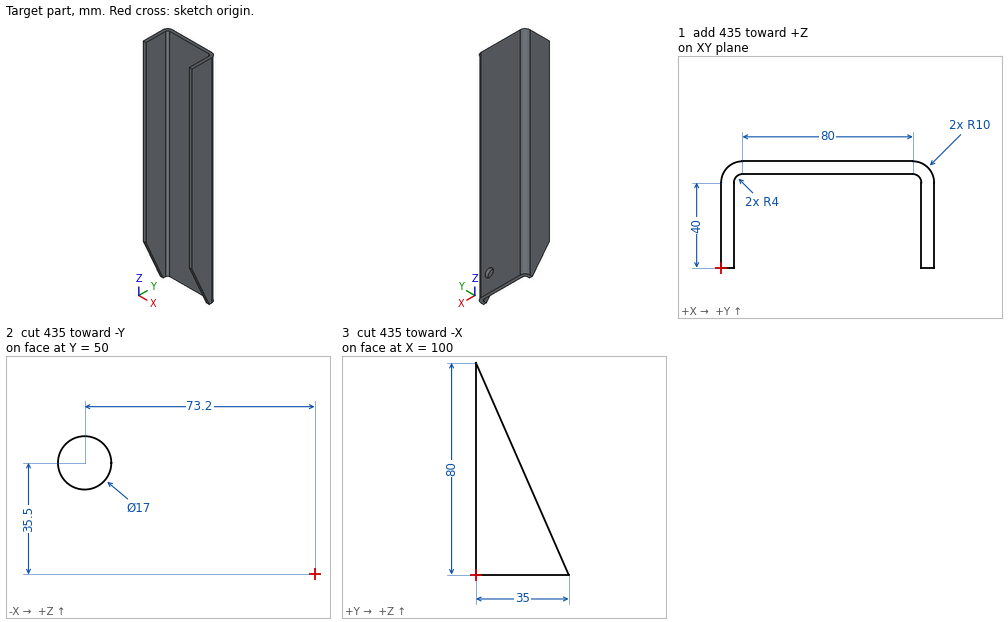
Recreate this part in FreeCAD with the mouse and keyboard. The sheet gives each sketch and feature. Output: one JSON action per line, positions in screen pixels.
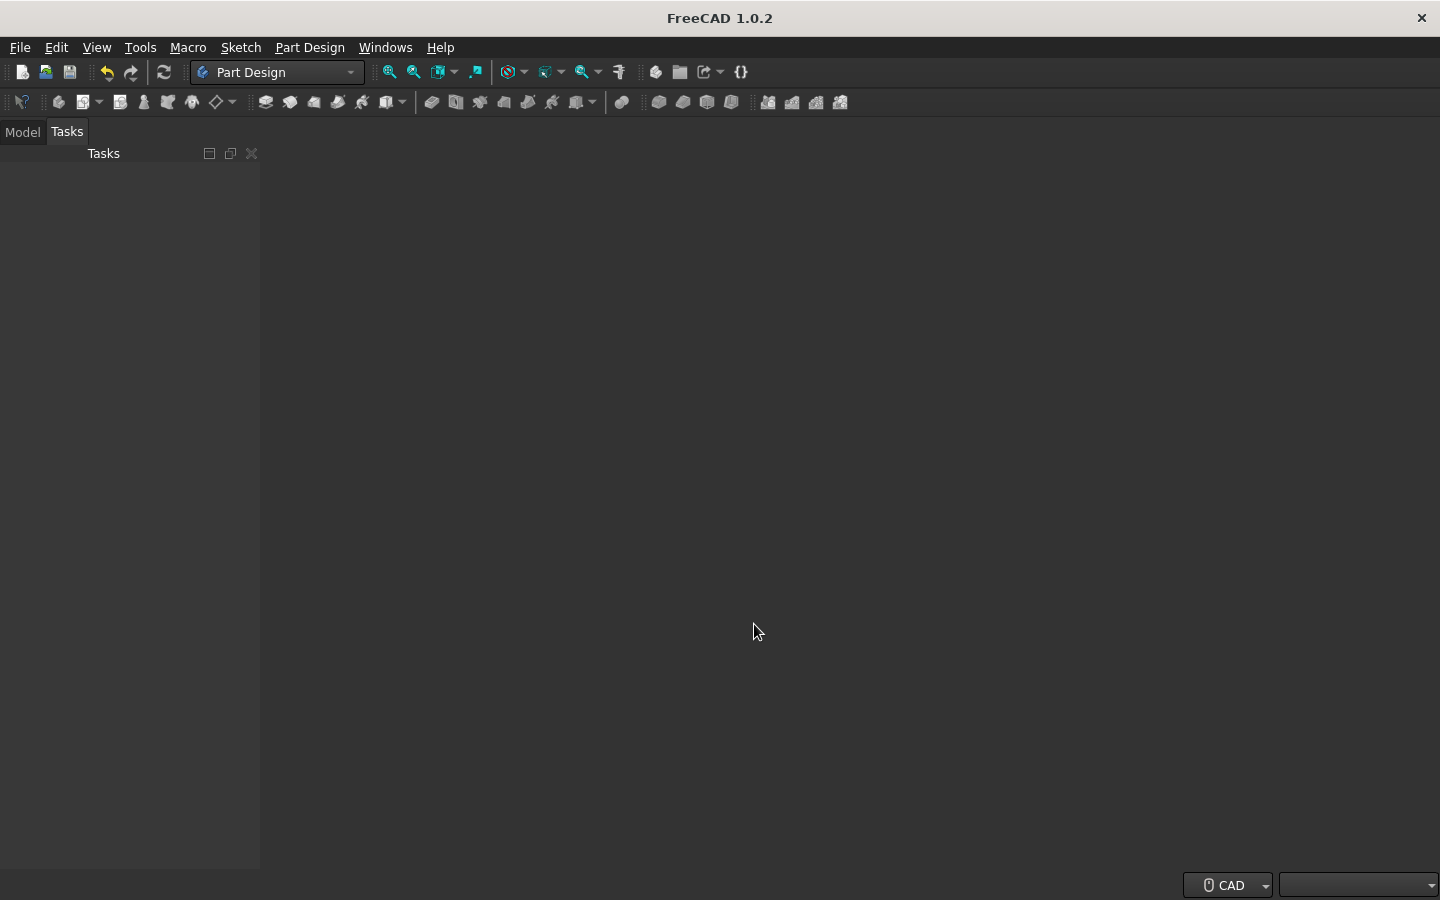
{"action": "left_click", "coordinate": [22, 72]}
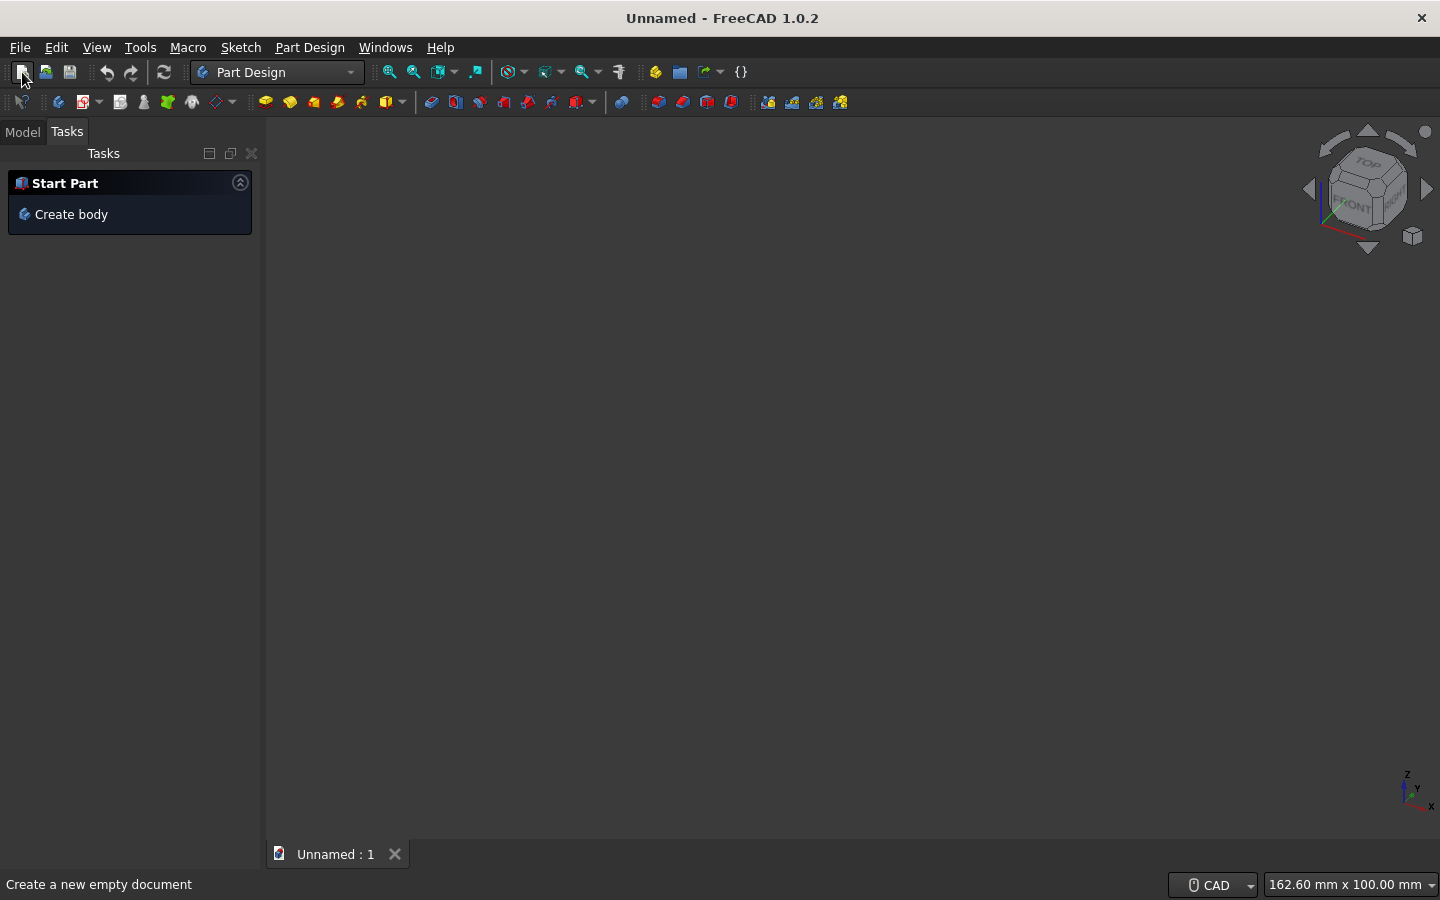
{"action": "left_click", "coordinate": [84, 102]}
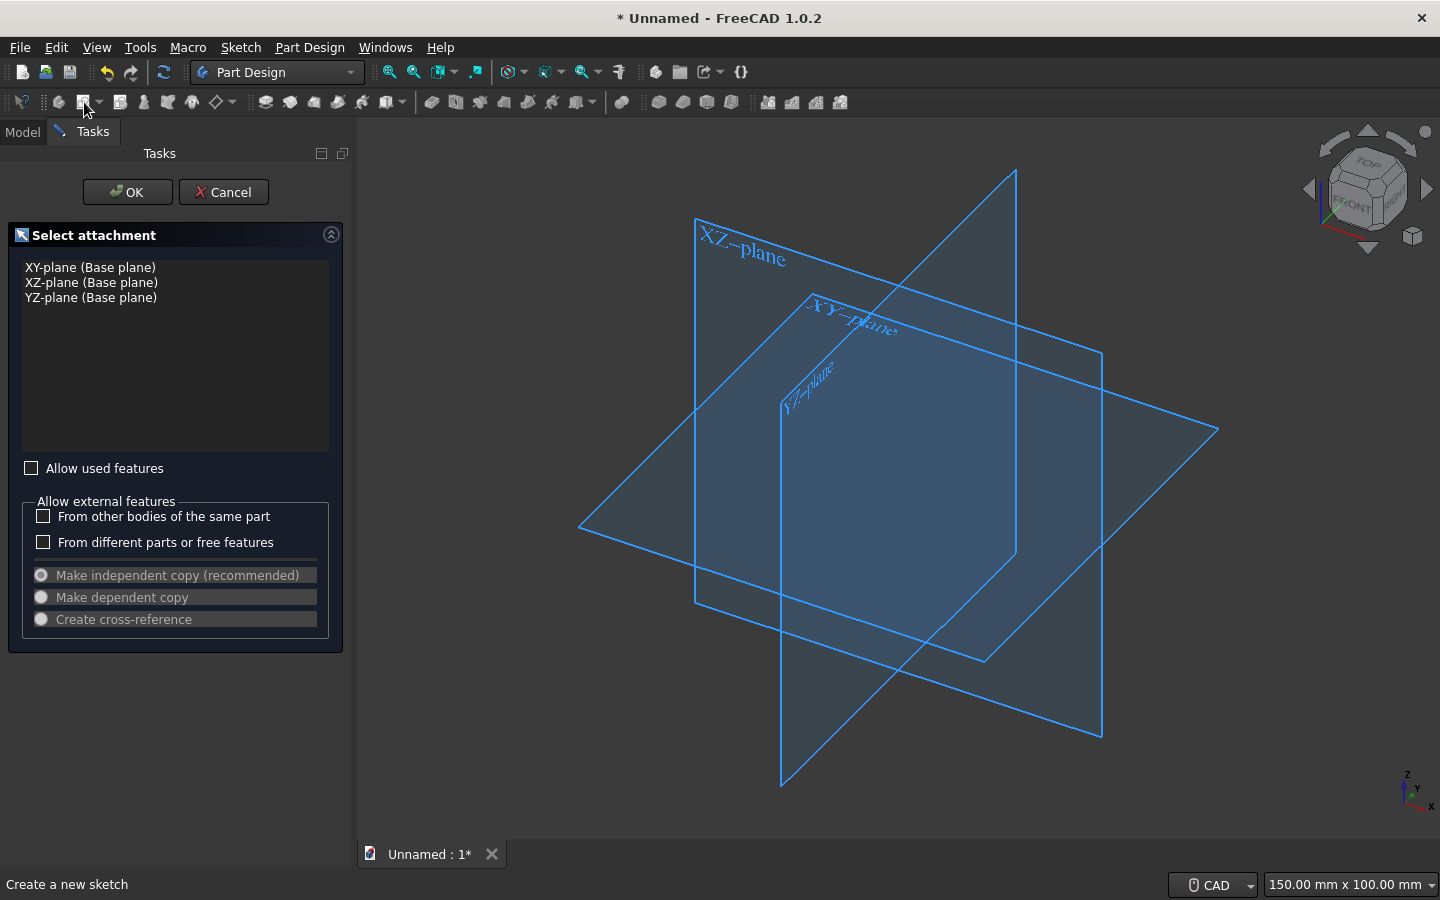
{"action": "left_click", "coordinate": [82, 268]}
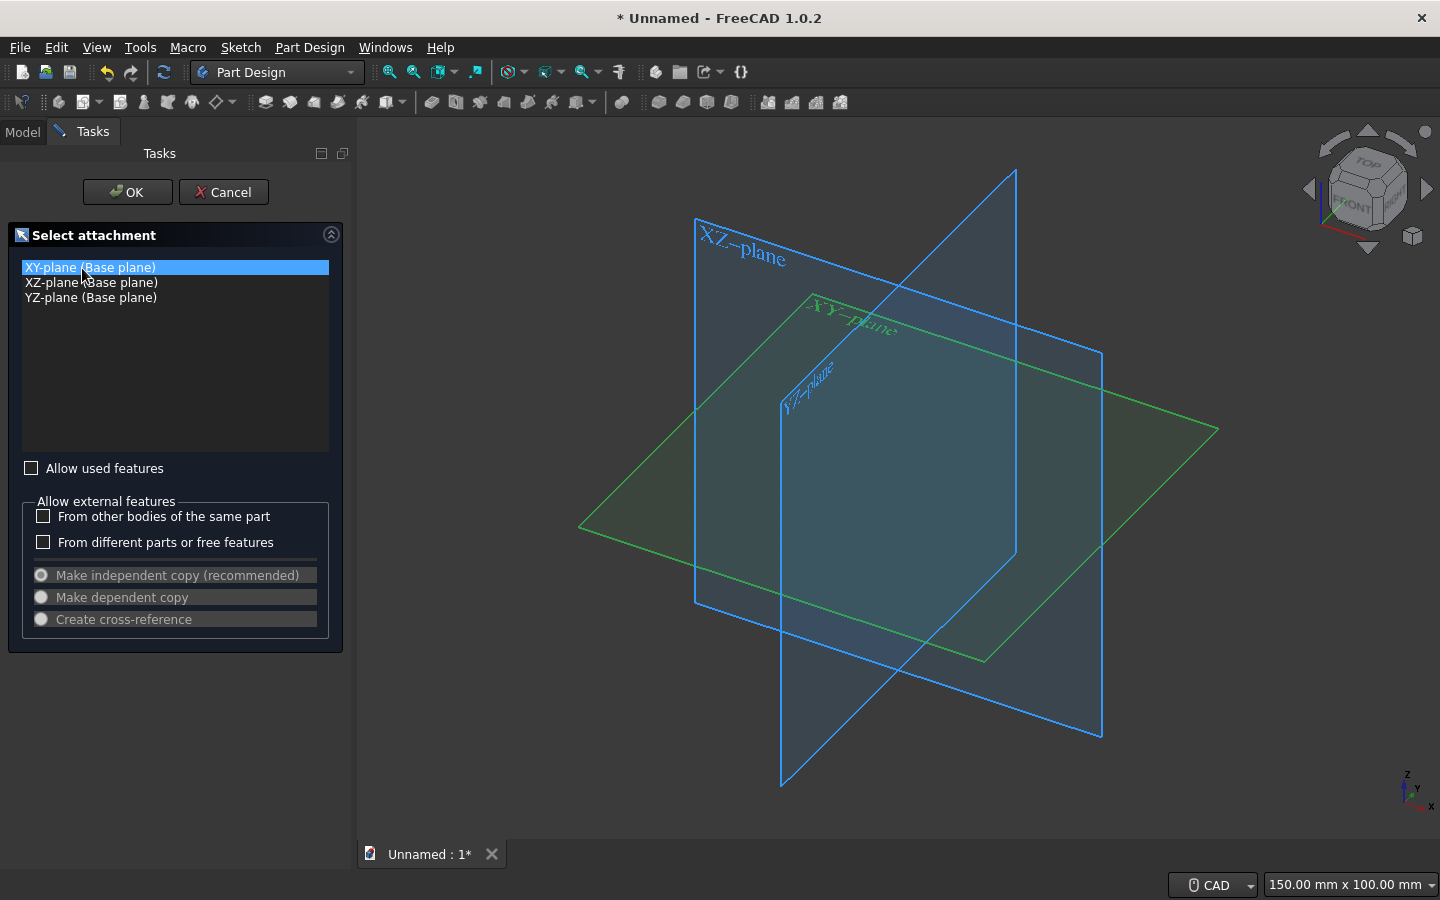
{"action": "left_click", "coordinate": [128, 192]}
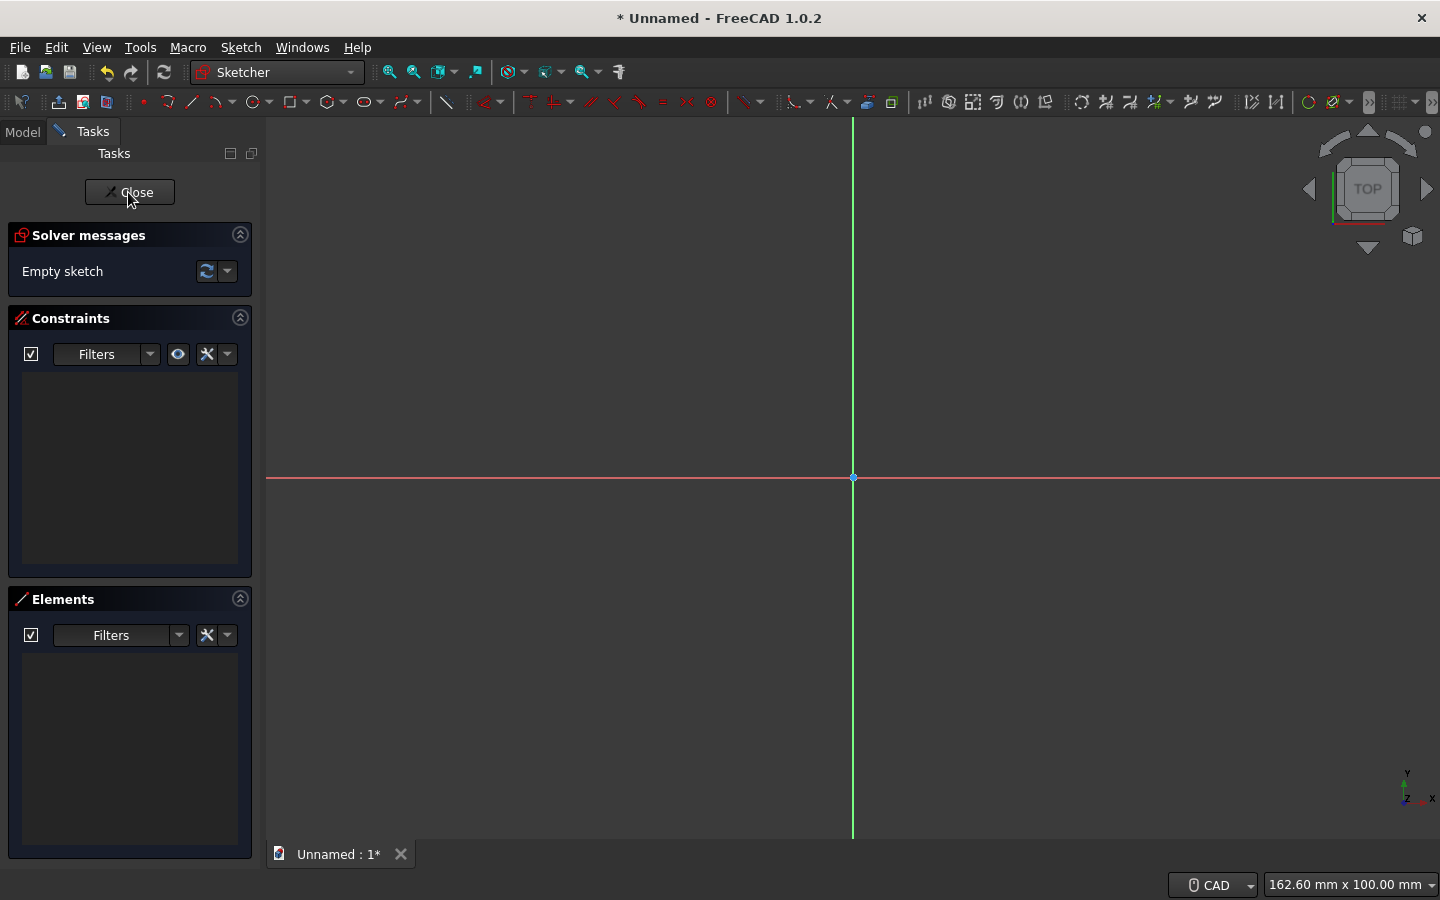
{"action": "scroll", "coordinate": [294, 811], "scroll_direction": "down", "scroll_amount": 2}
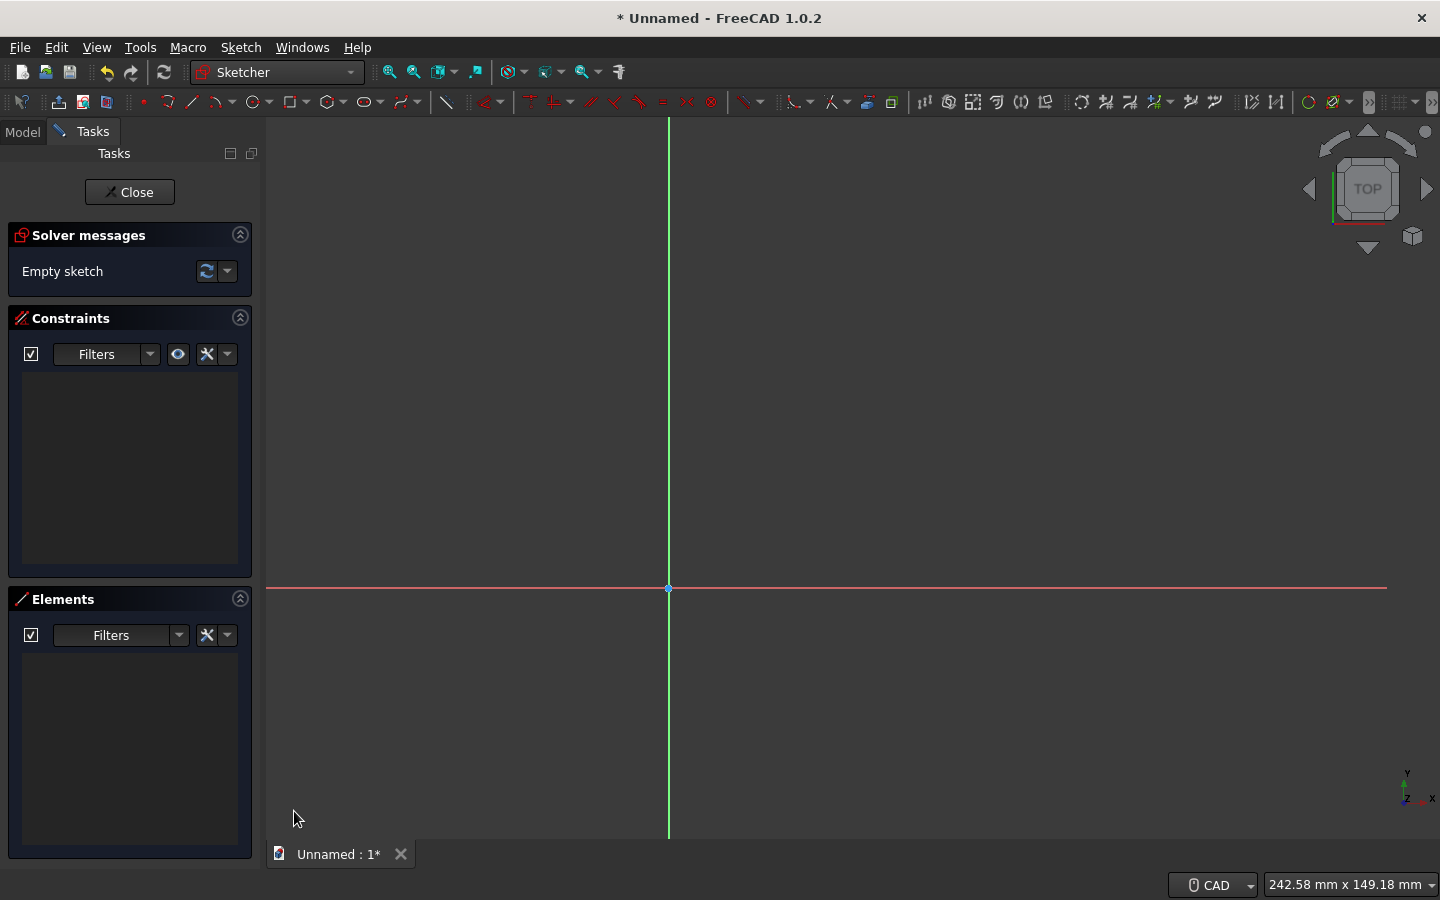
{"action": "scroll", "coordinate": [1167, 445], "scroll_direction": "up", "scroll_amount": 2}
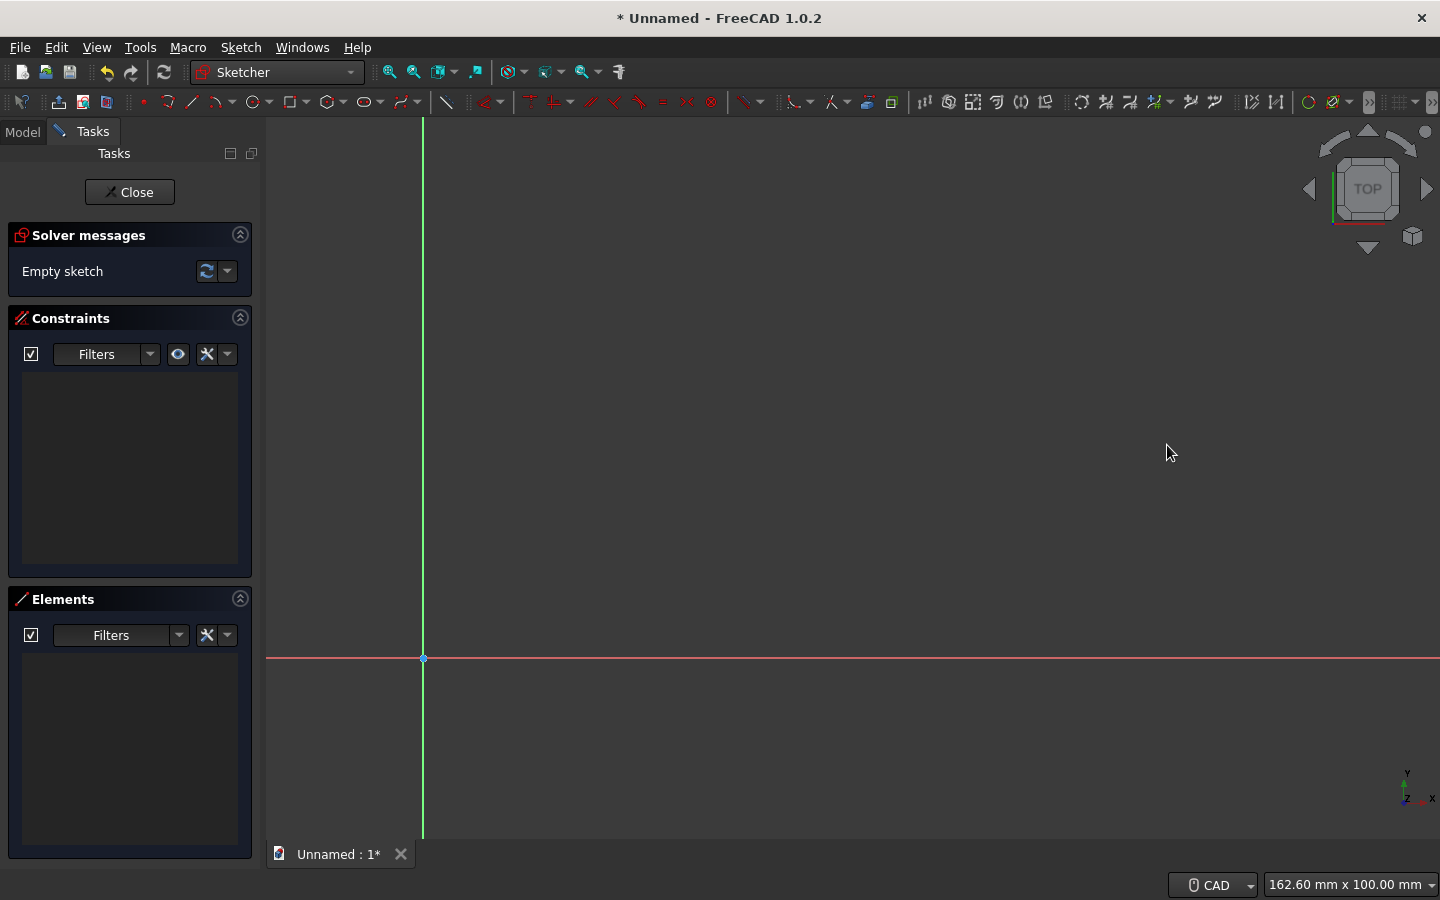
{"action": "left_click", "coordinate": [168, 102]}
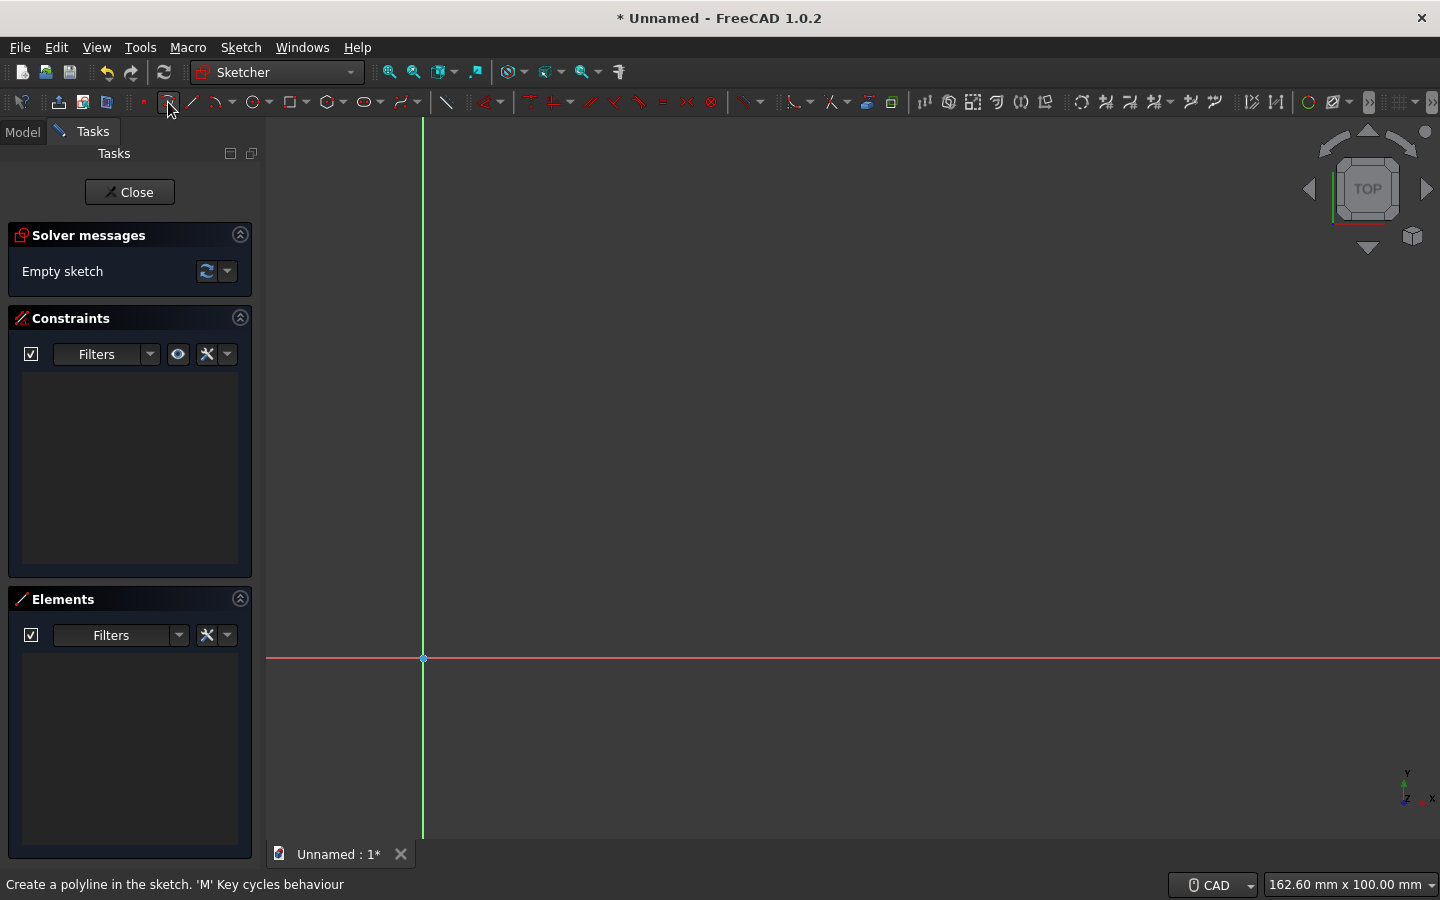
{"action": "left_click", "coordinate": [423, 369]}
{"action": "left_click", "coordinate": [423, 658]}
{"action": "left_click", "coordinate": [467, 649]}
{"action": "left_click", "coordinate": [467, 369]}
{"action": "right_click", "coordinate": [467, 369]}